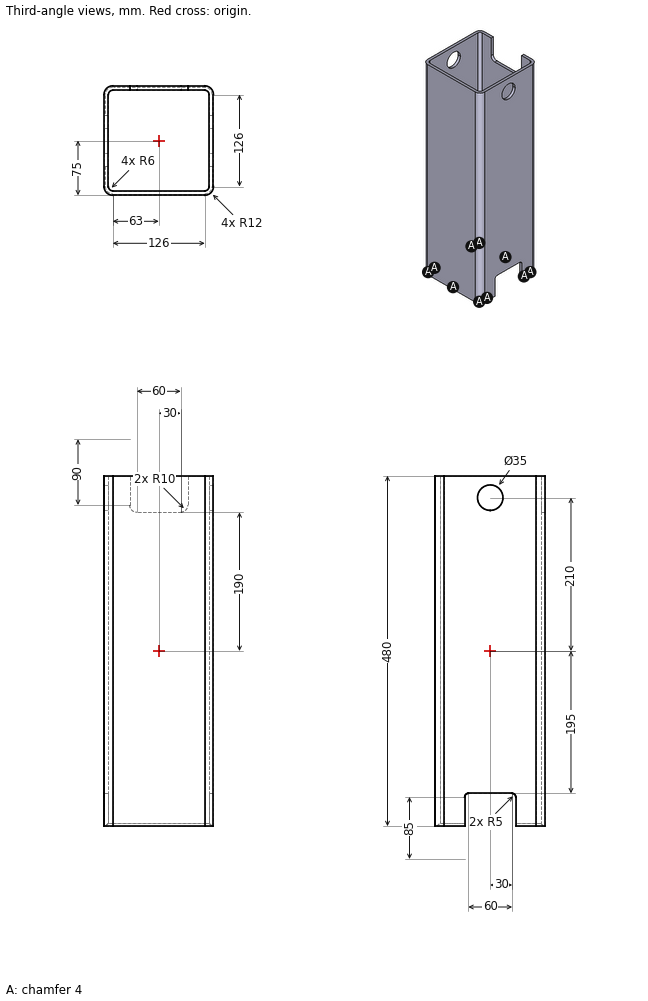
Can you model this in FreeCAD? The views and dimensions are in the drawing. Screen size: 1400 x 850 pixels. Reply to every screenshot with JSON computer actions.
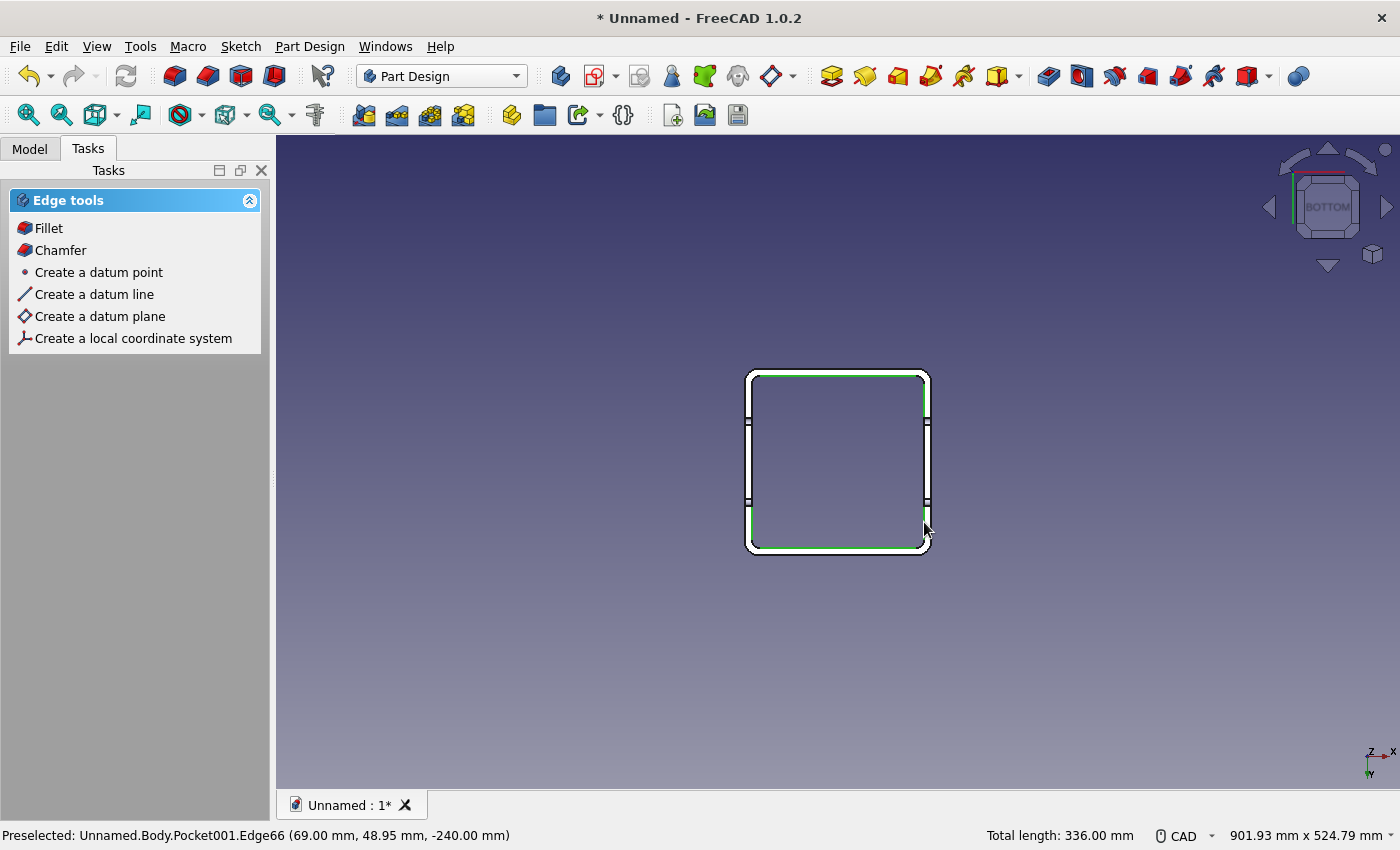
{"action": "left_click", "coordinate": [752, 400], "text": "ctrl"}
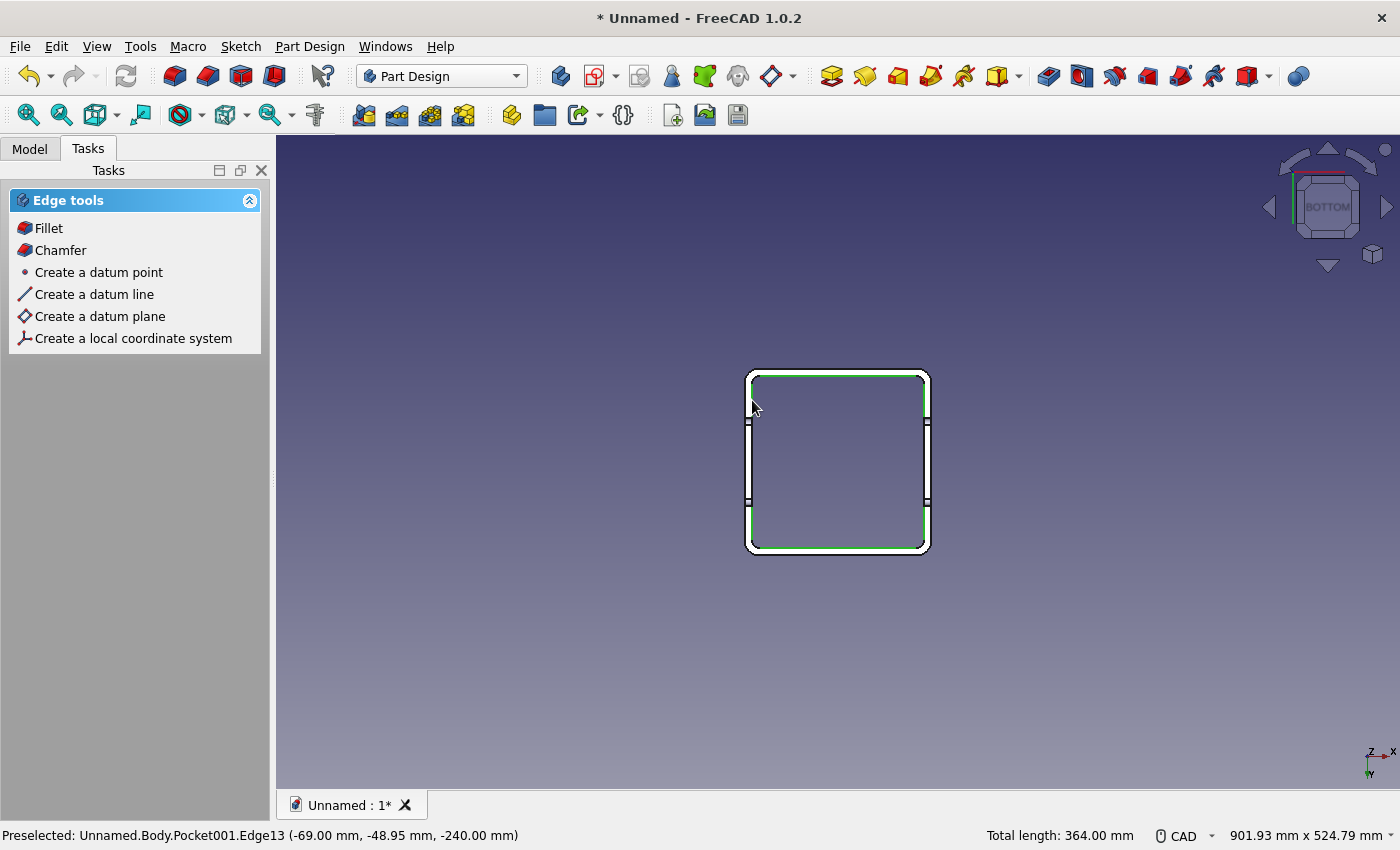
{"action": "scroll", "coordinate": [754, 545], "scroll_direction": "up", "scroll_amount": 7}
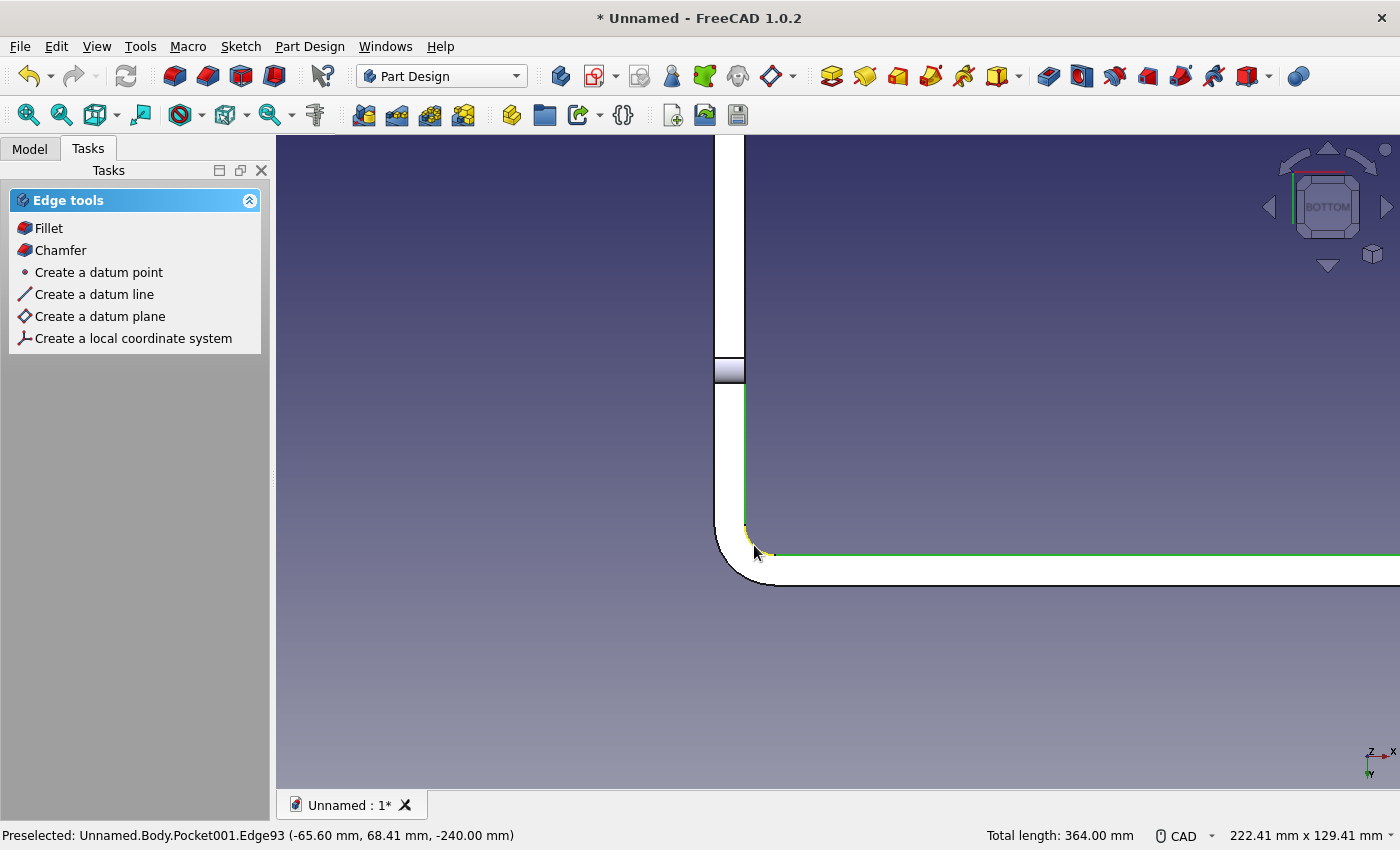
{"action": "left_click", "coordinate": [754, 545], "text": "ctrl"}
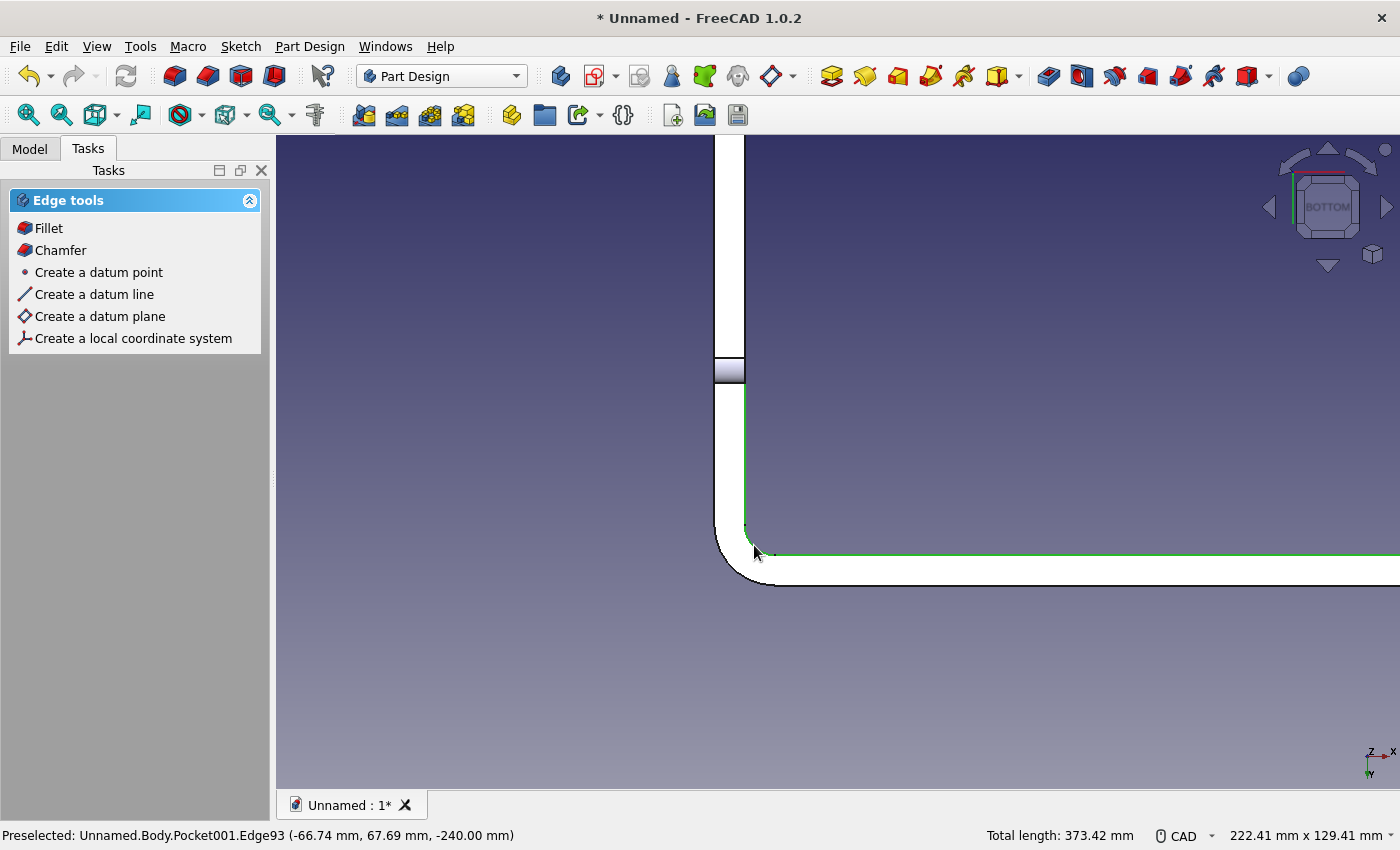
{"action": "key", "text": "v f"}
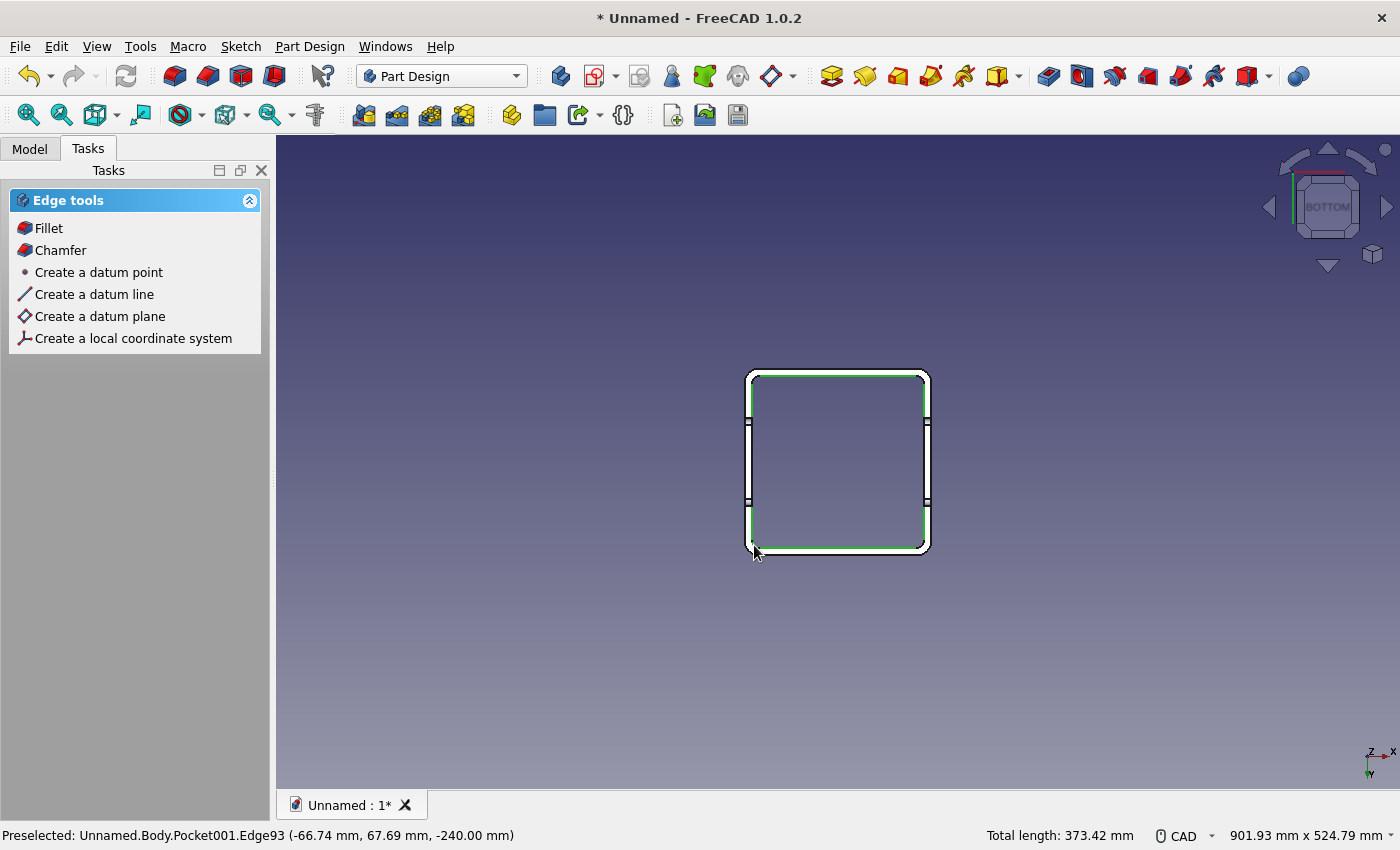
{"action": "key", "text": "4"}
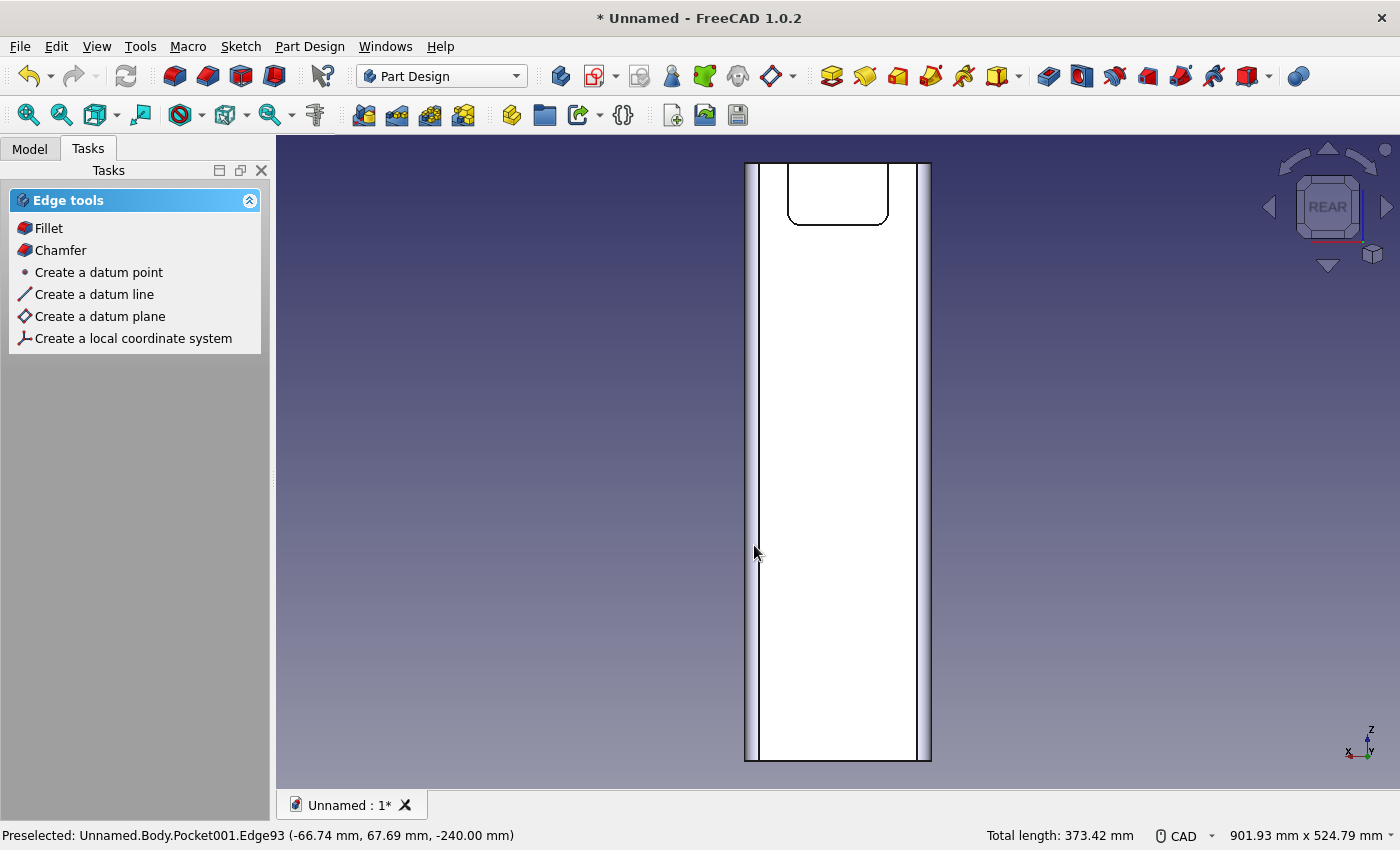
{"action": "scroll", "coordinate": [922, 760], "scroll_direction": "up", "scroll_amount": 7}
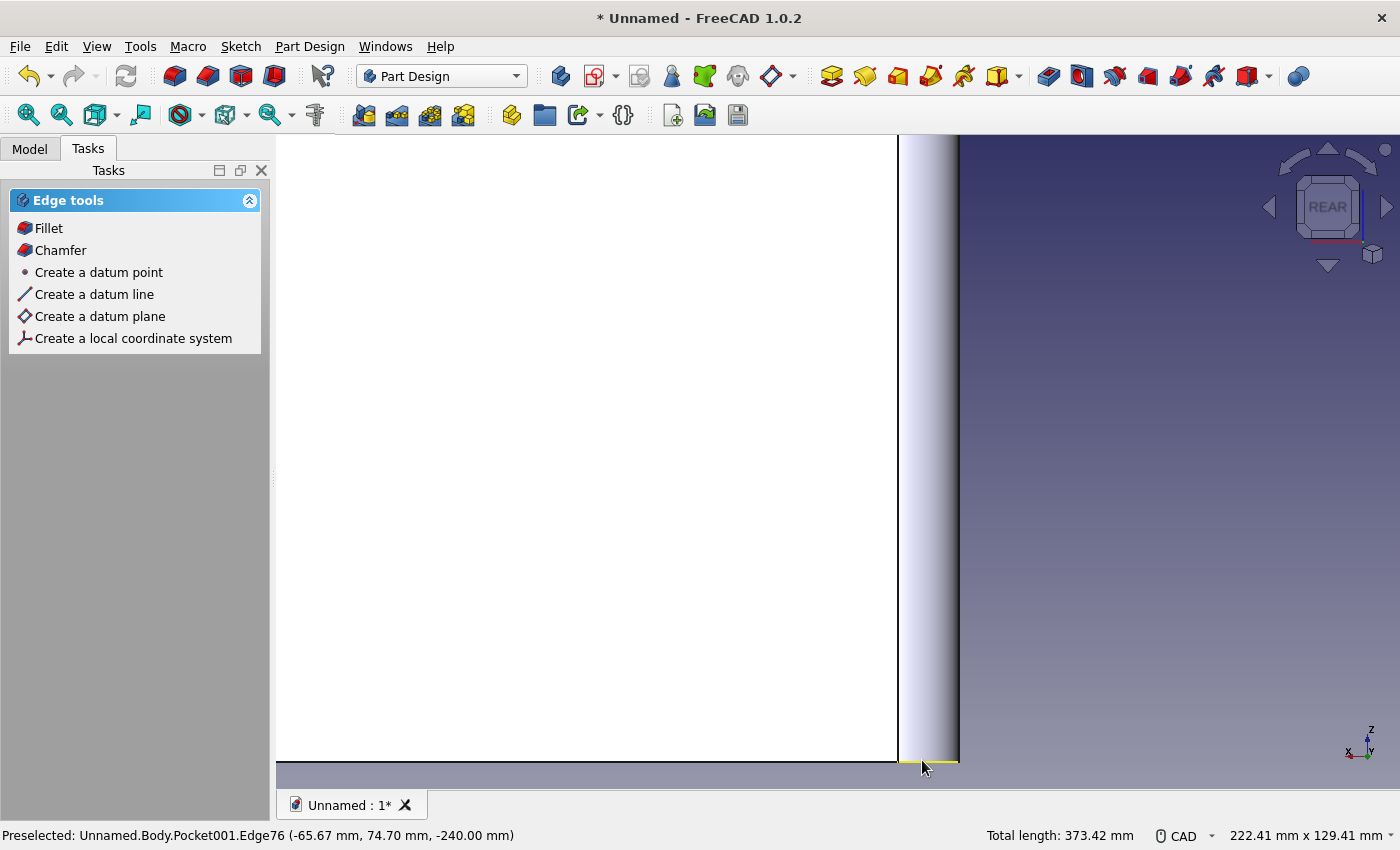
{"action": "key", "text": "v f"}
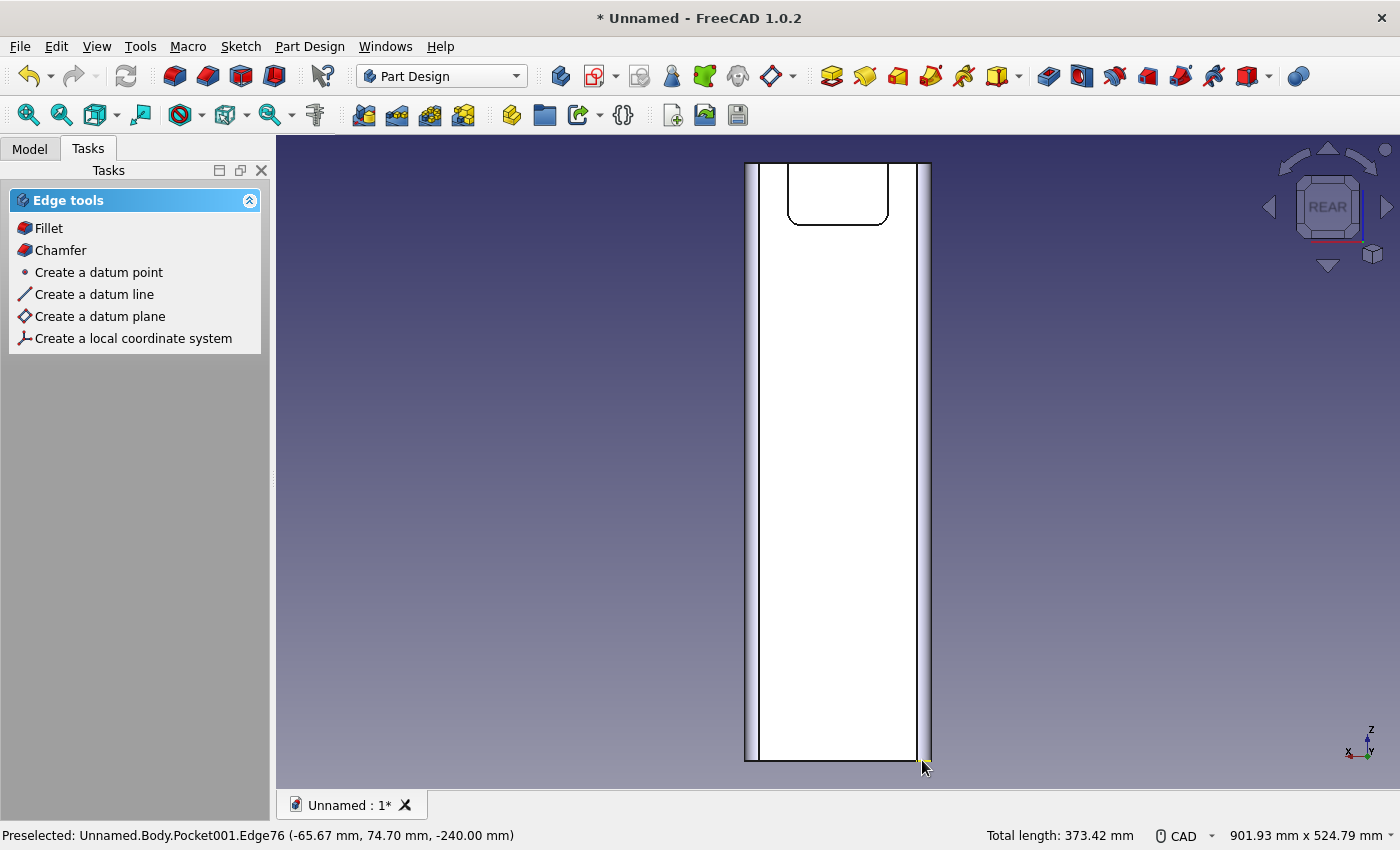
{"action": "key", "text": "6"}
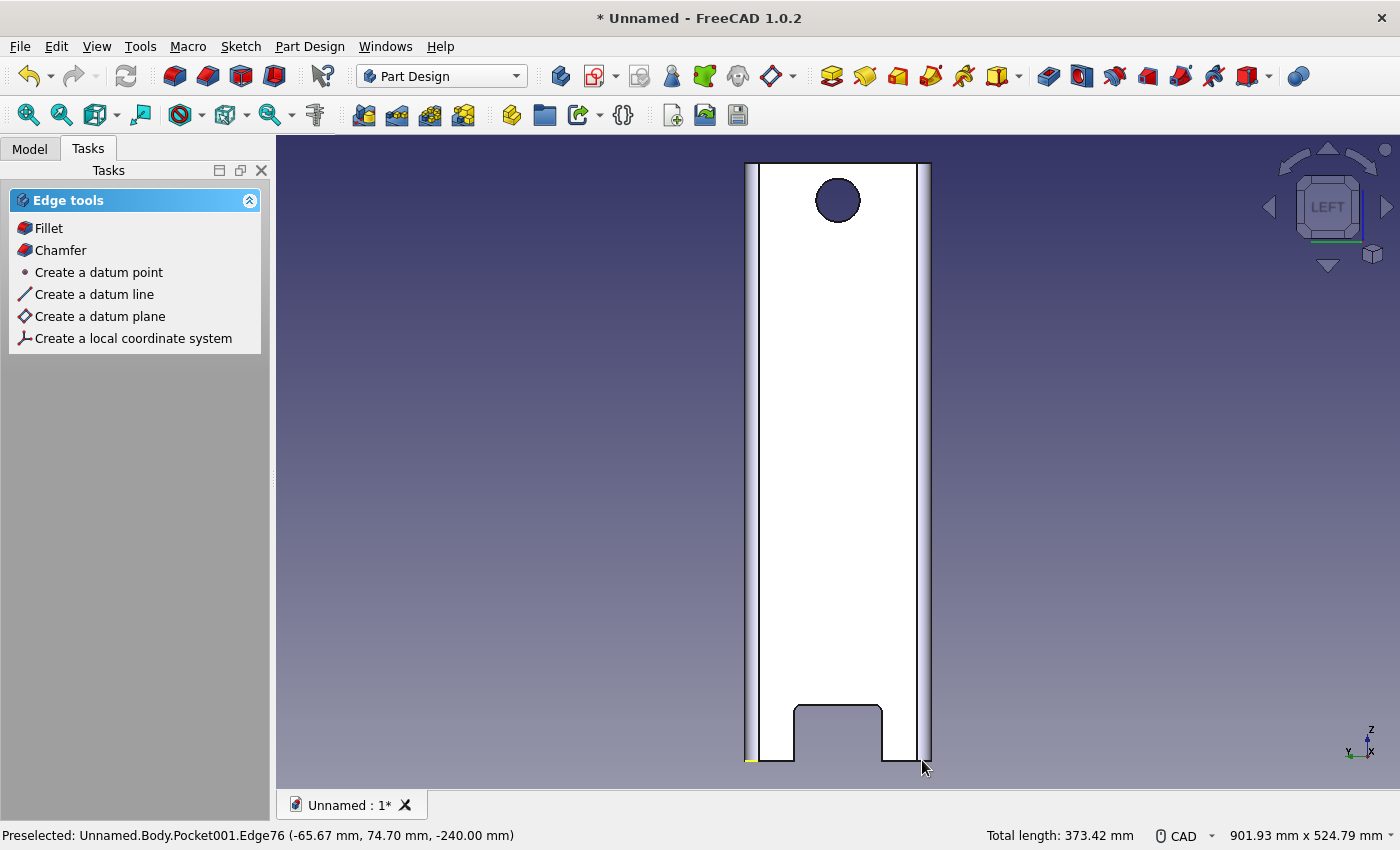
{"action": "scroll", "coordinate": [922, 760], "scroll_direction": "up", "scroll_amount": 7}